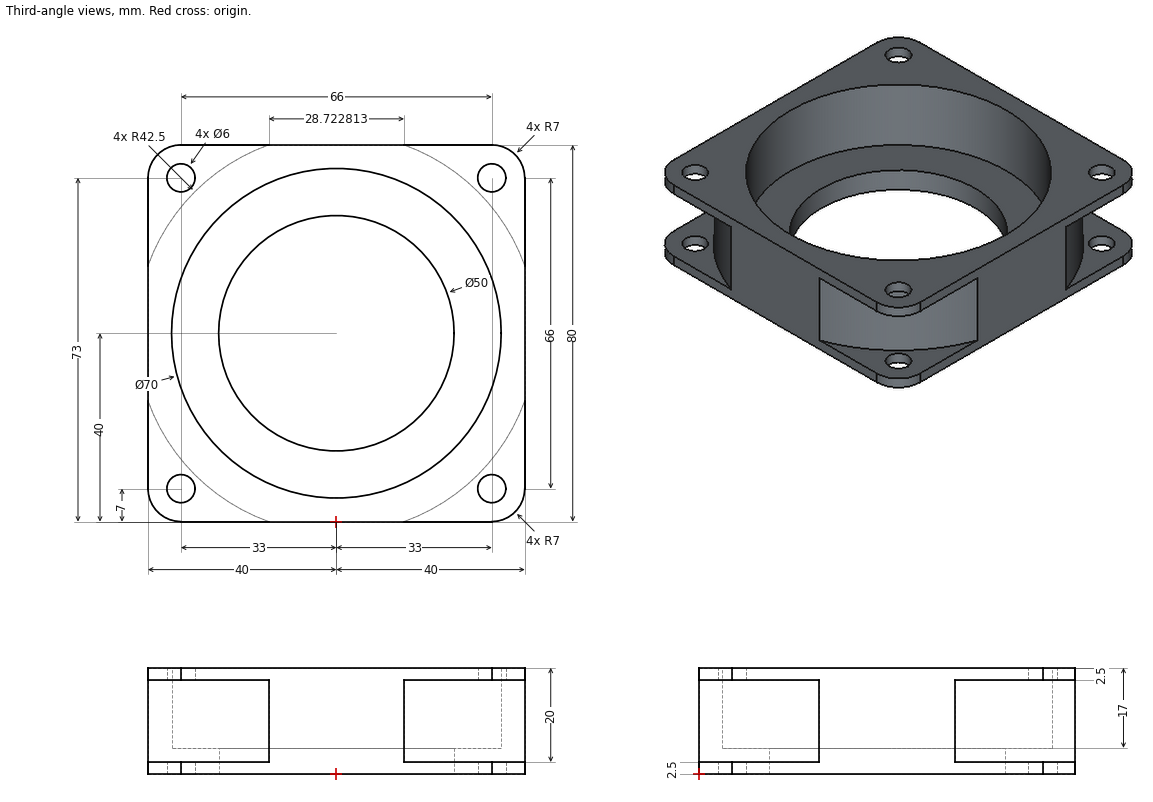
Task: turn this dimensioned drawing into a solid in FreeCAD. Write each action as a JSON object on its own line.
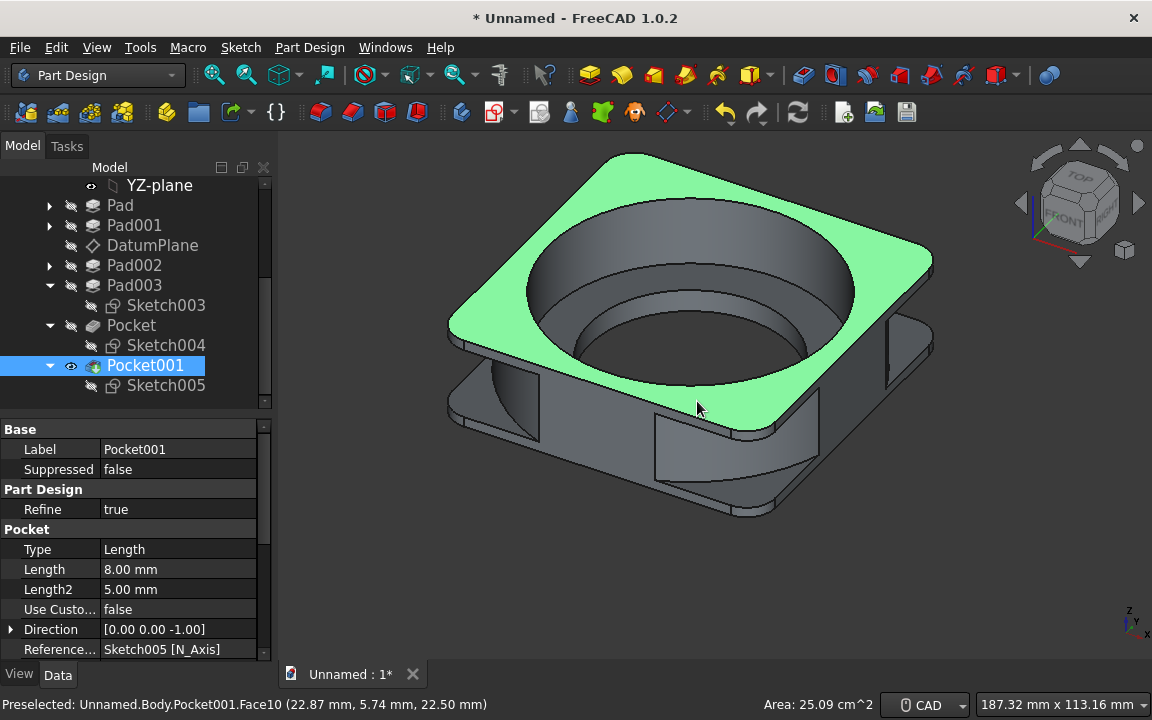
{"action": "left_click", "coordinate": [494, 112]}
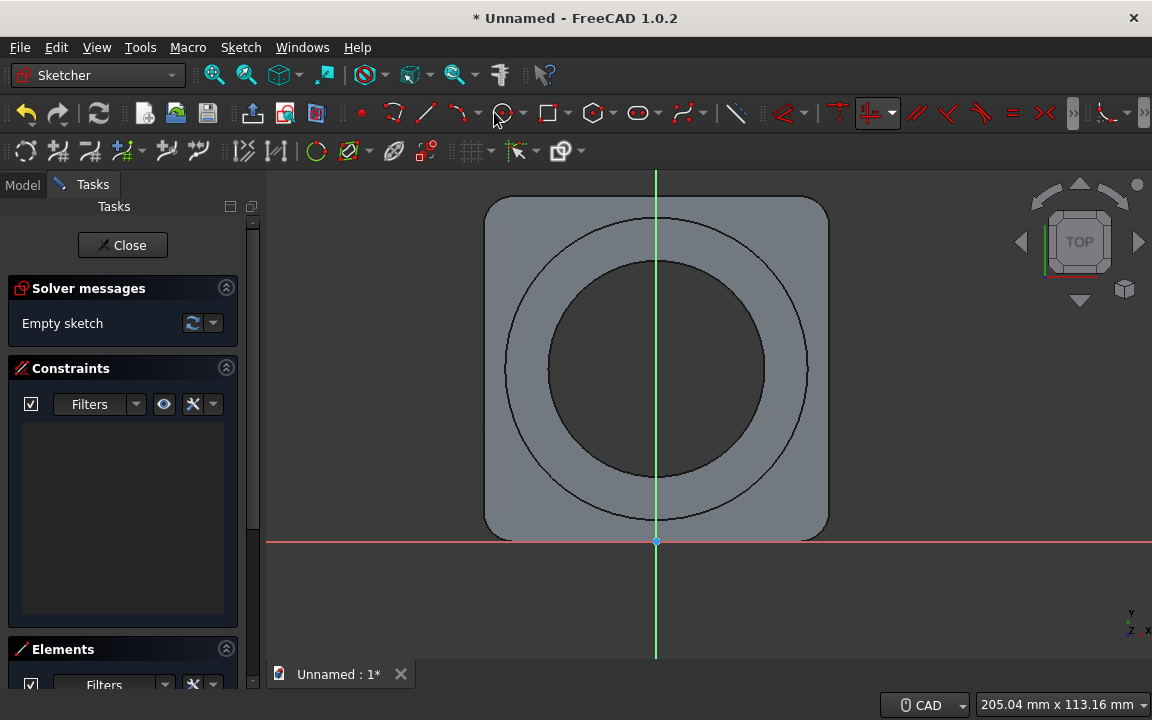
{"action": "scroll", "coordinate": [568, 582], "scroll_direction": "down", "scroll_amount": 1}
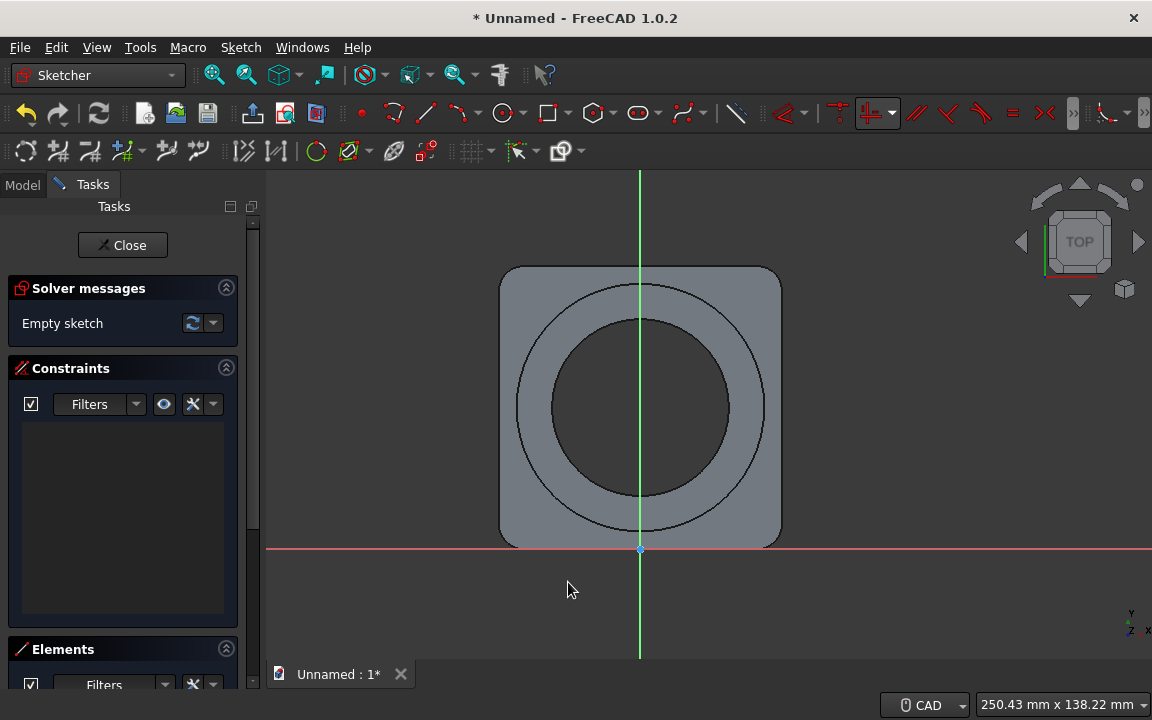
{"action": "key", "text": "g c"}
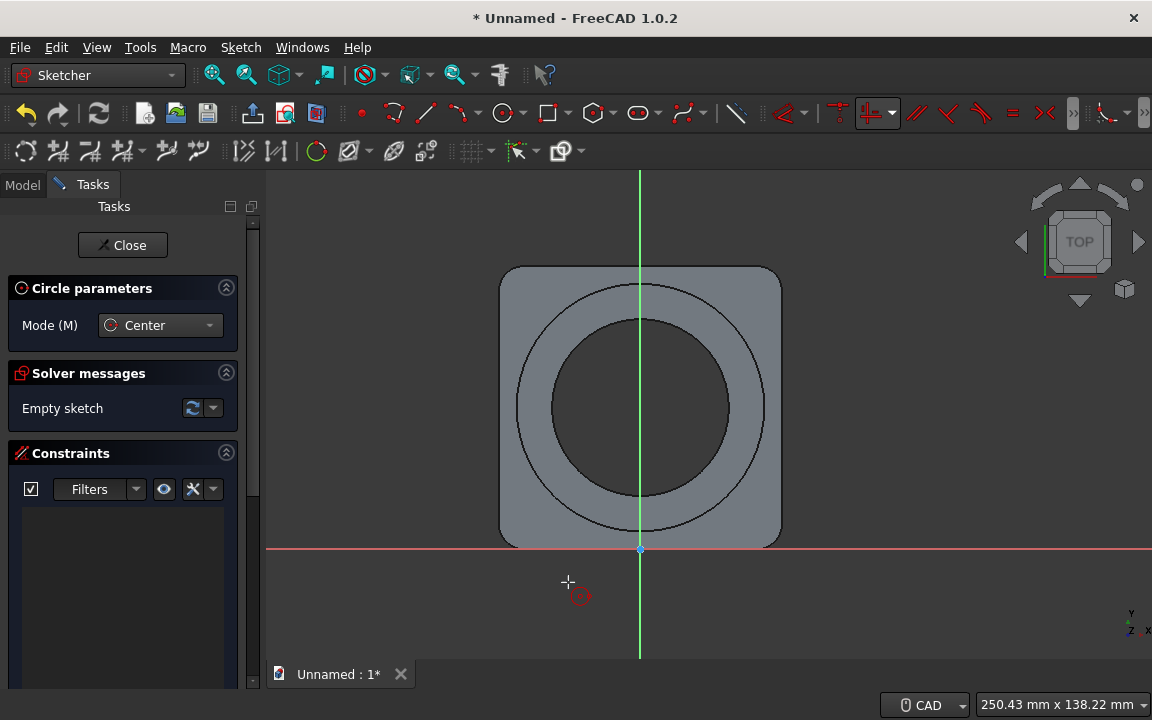
{"action": "scroll", "coordinate": [524, 291], "scroll_direction": "up", "scroll_amount": 4}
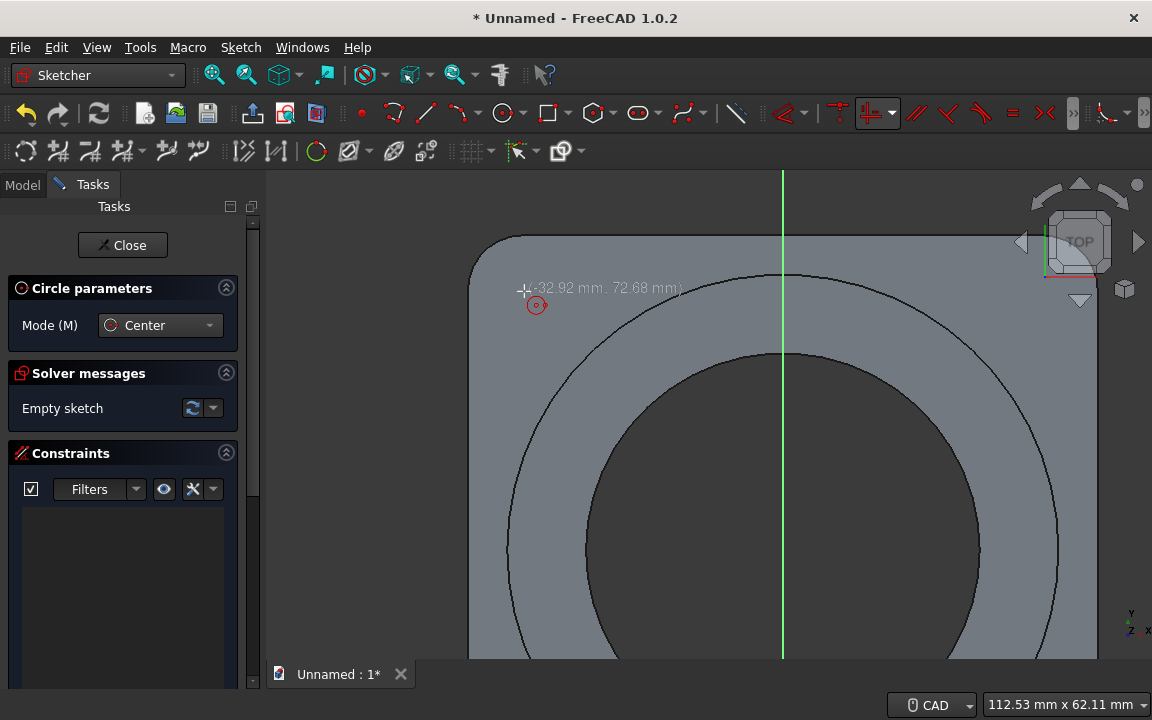
{"action": "left_click", "coordinate": [523, 290]}
{"action": "mouse_move", "coordinate": [540, 274]}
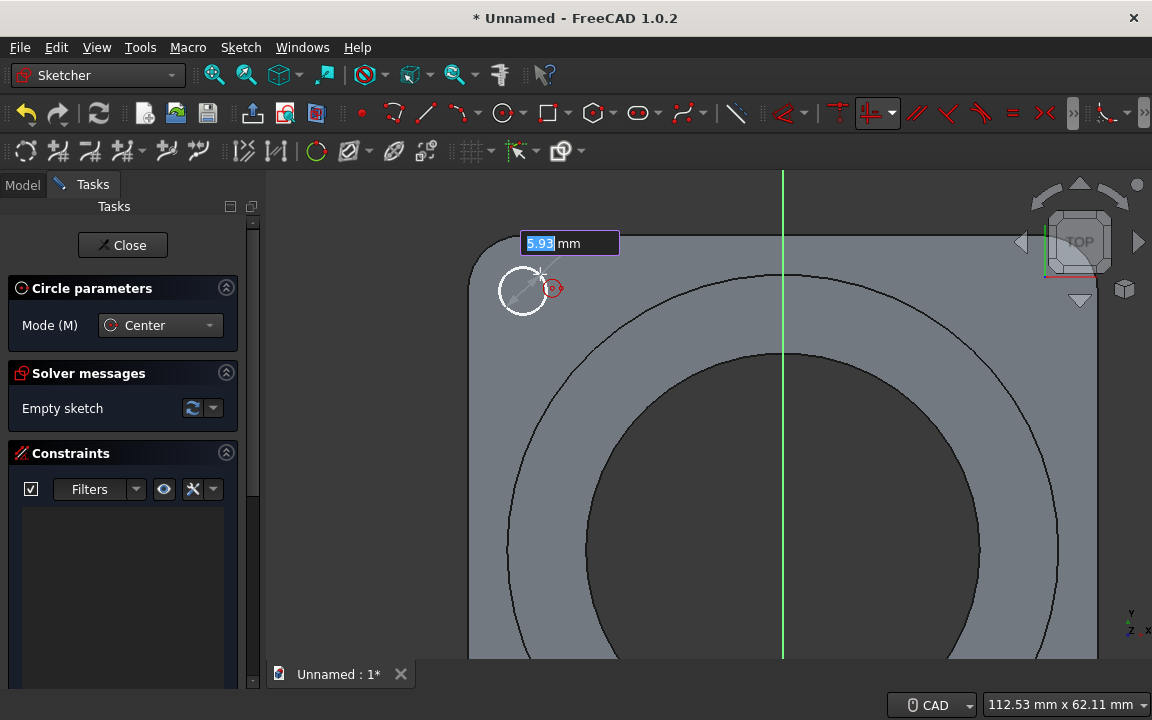
{"action": "type", "text": "6"}
{"action": "key", "text": "Return"}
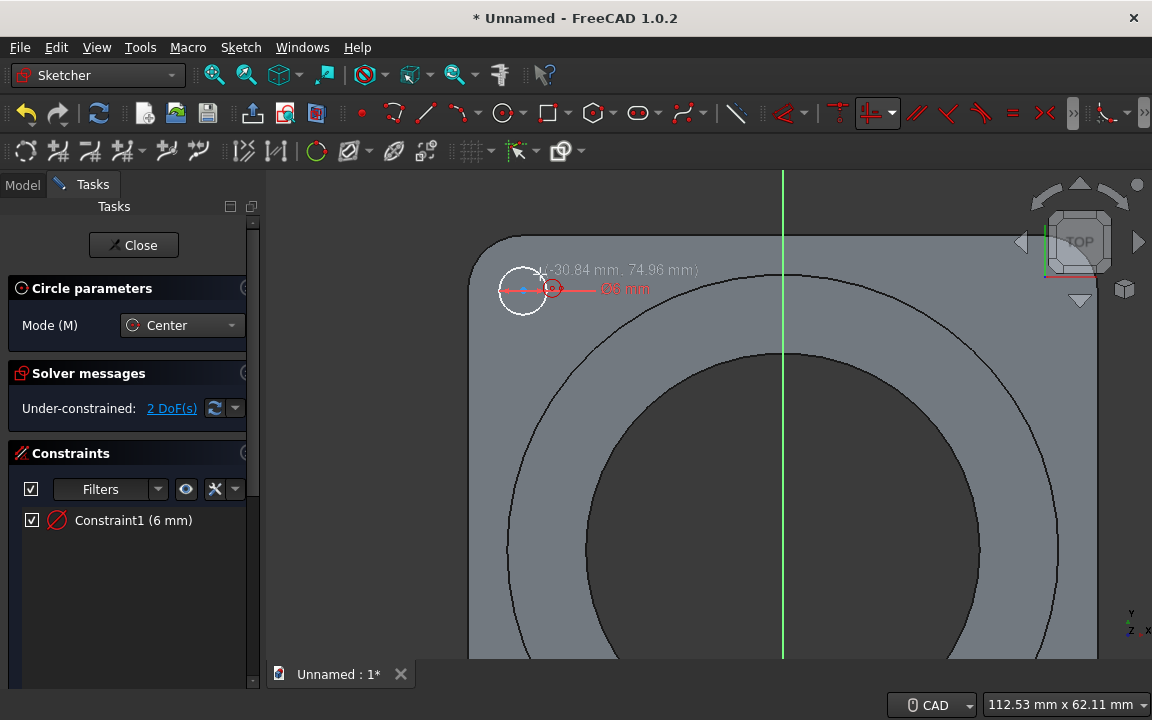
{"action": "scroll", "coordinate": [467, 230], "scroll_direction": "down", "scroll_amount": 3}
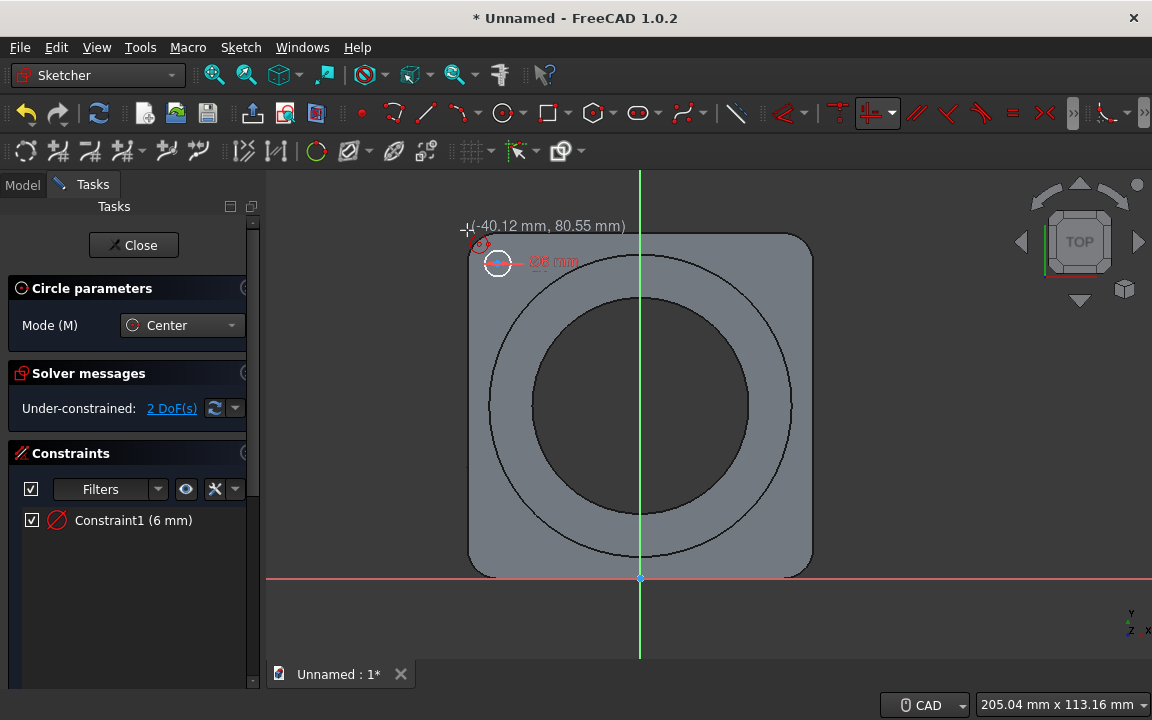
{"action": "scroll", "coordinate": [783, 263], "scroll_direction": "up", "scroll_amount": 3}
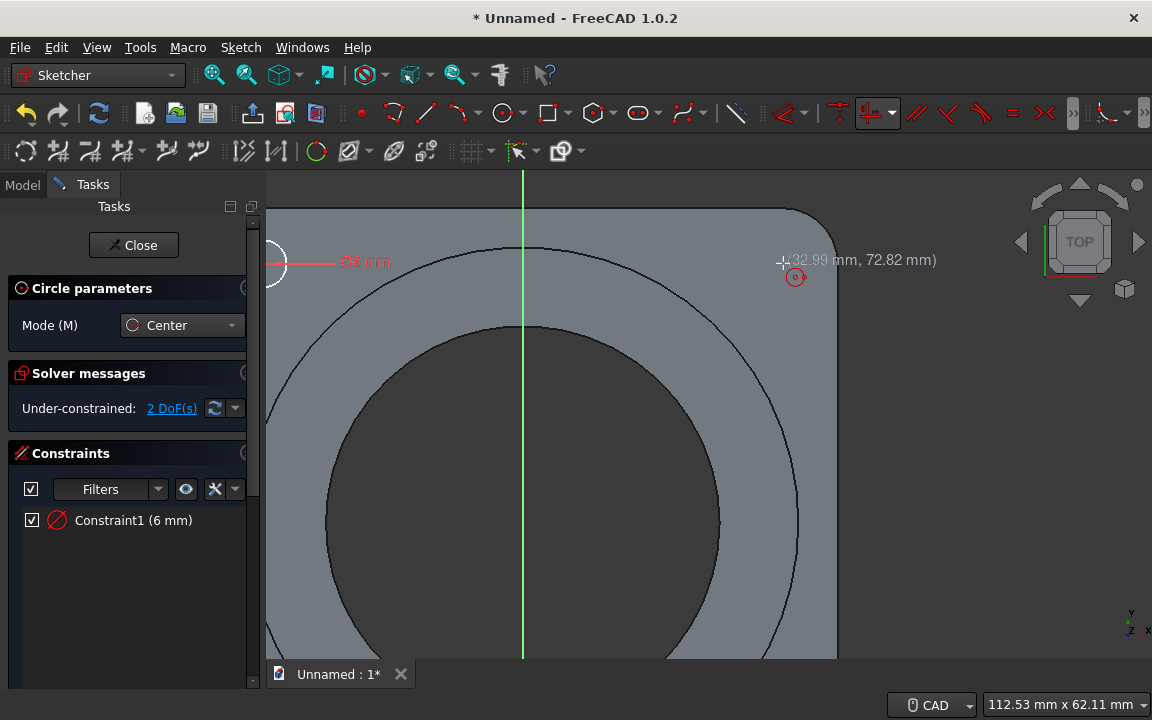
{"action": "left_click", "coordinate": [783, 263]}
{"action": "mouse_move", "coordinate": [799, 247]}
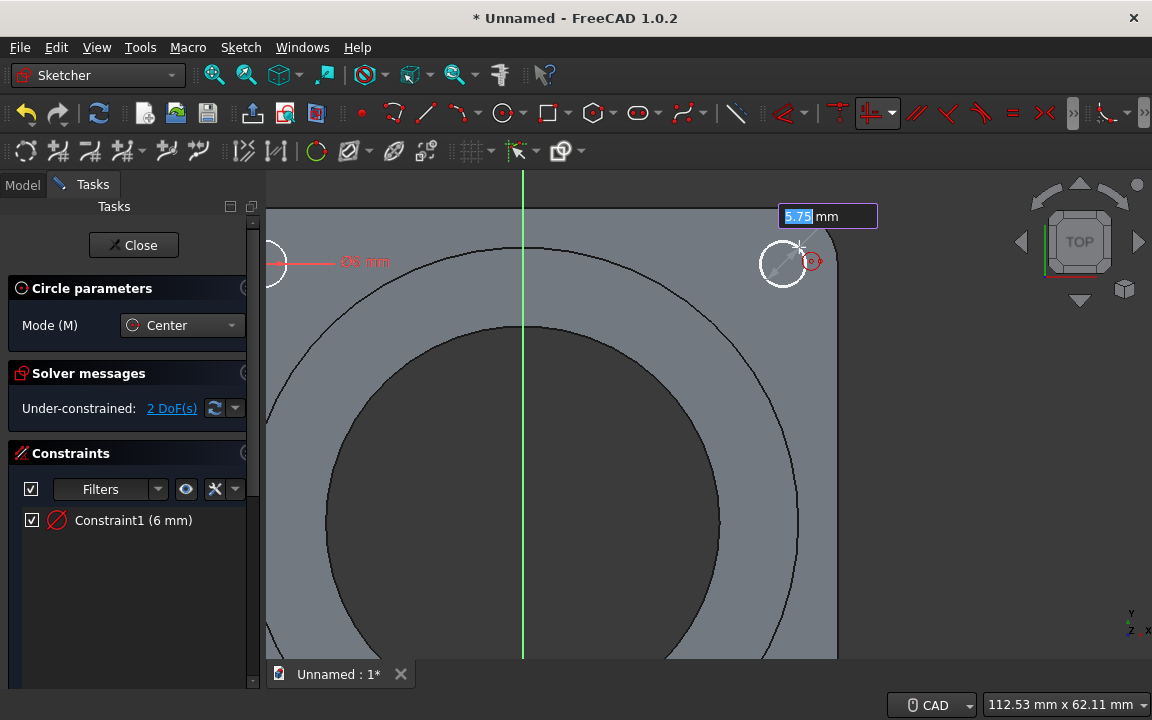
{"action": "type", "text": "6"}
{"action": "key", "text": "Return"}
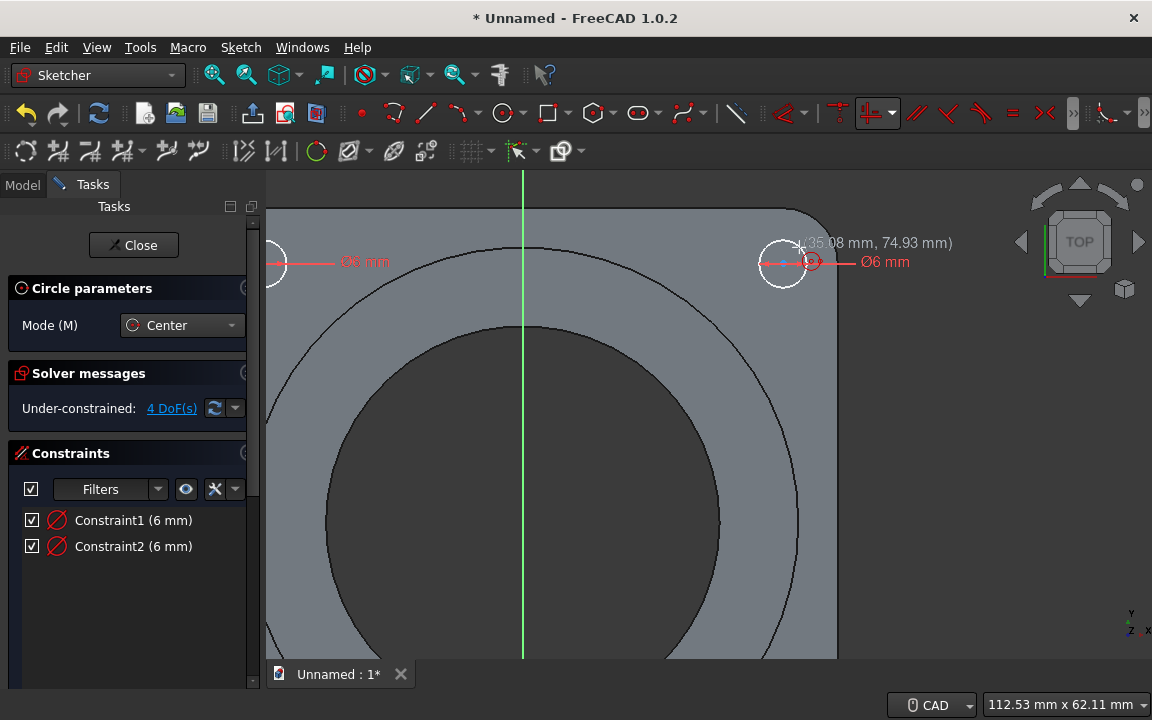
{"action": "scroll", "coordinate": [784, 263], "scroll_direction": "down", "scroll_amount": 3}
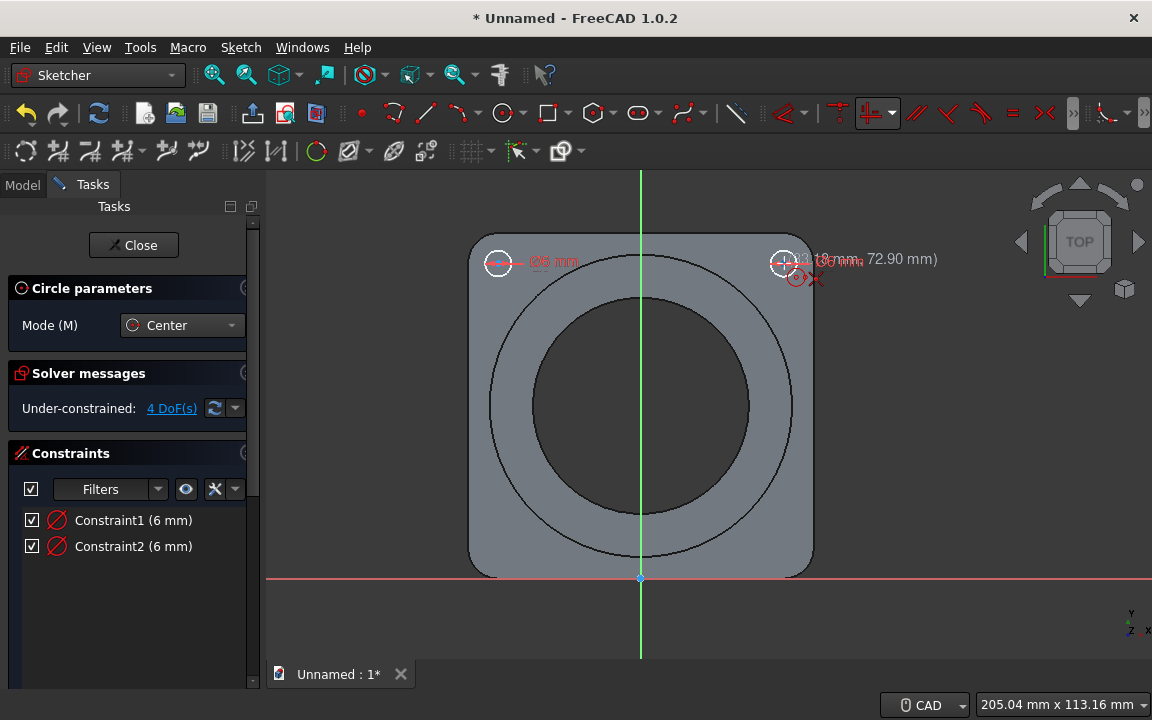
{"action": "scroll", "coordinate": [498, 548], "scroll_direction": "up", "scroll_amount": 3}